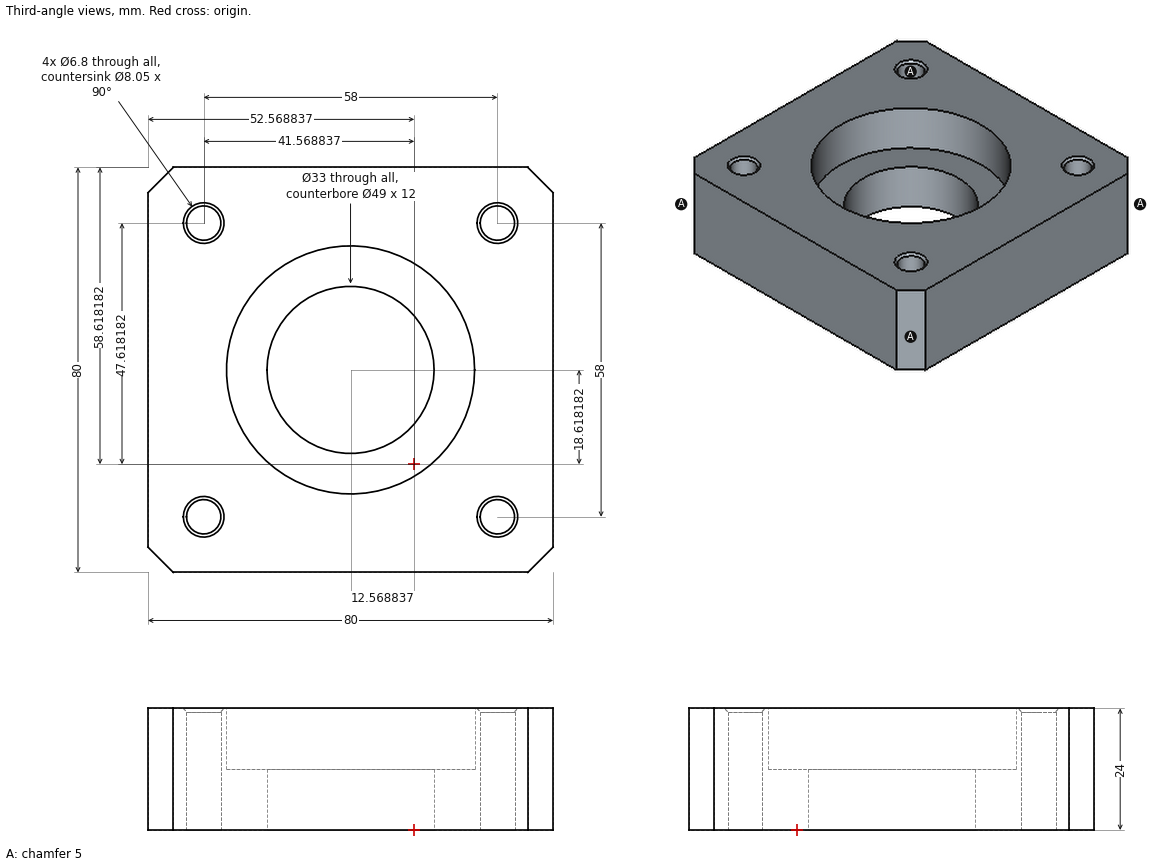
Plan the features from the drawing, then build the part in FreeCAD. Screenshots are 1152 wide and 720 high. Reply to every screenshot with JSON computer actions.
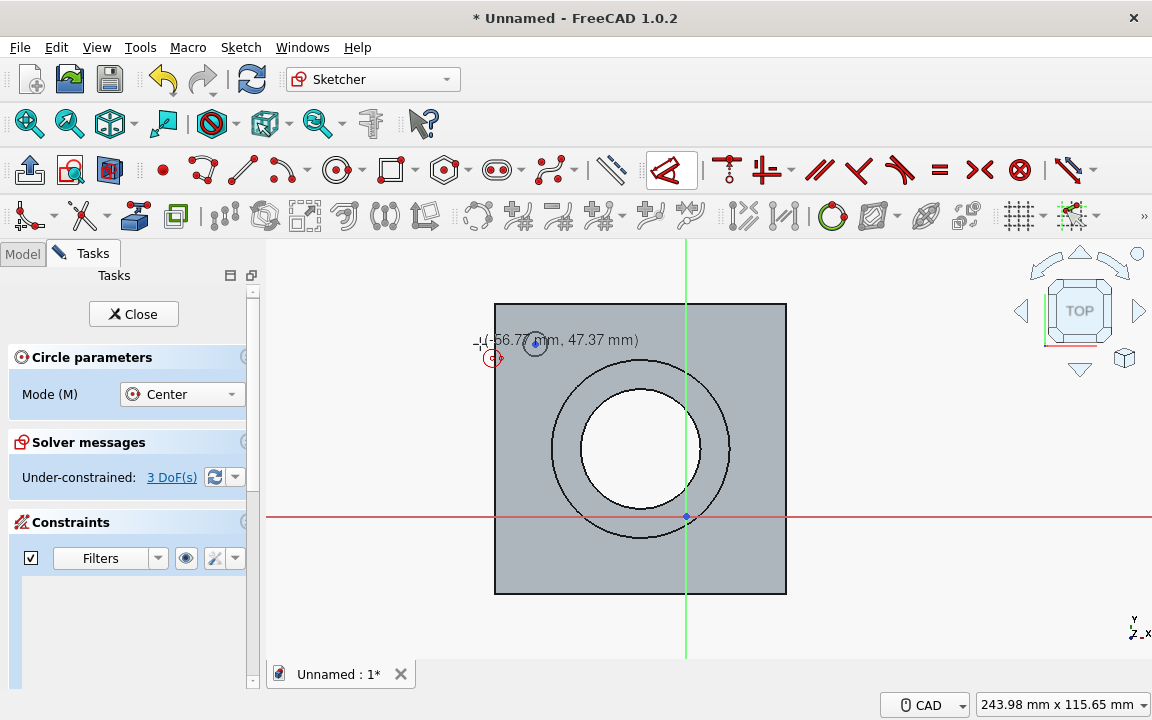
{"action": "scroll", "coordinate": [746, 344], "scroll_direction": "up", "scroll_amount": 4}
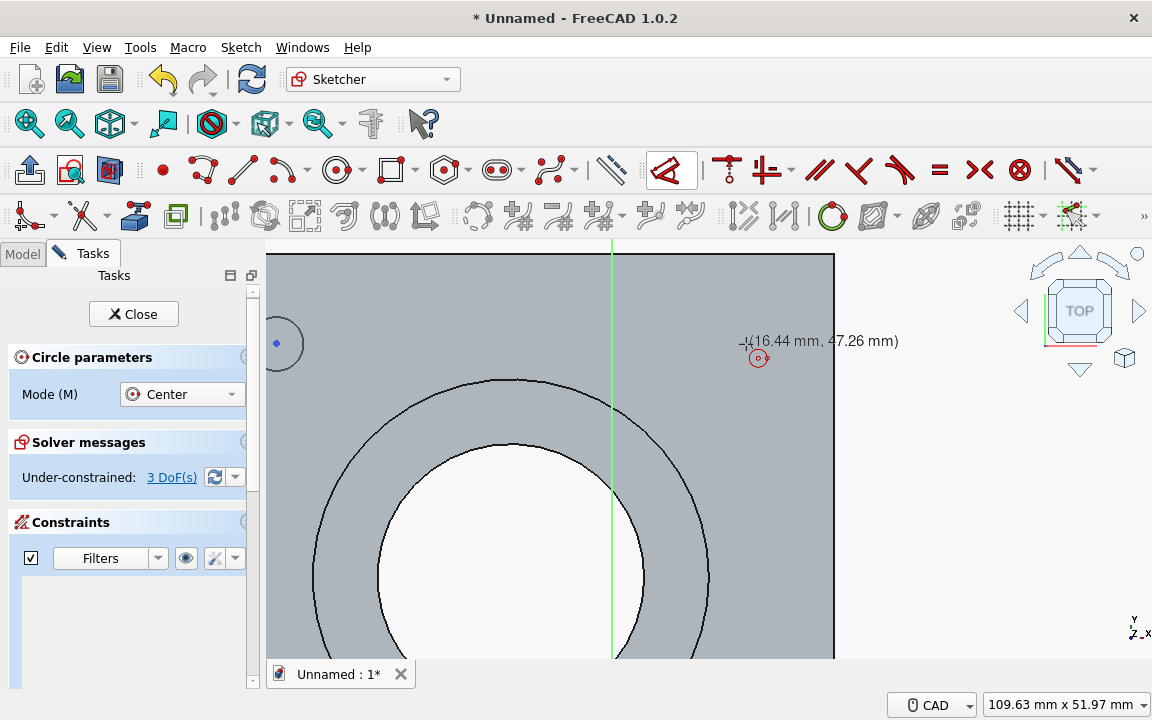
{"action": "left_click", "coordinate": [745, 343]}
{"action": "left_click", "coordinate": [765, 324]}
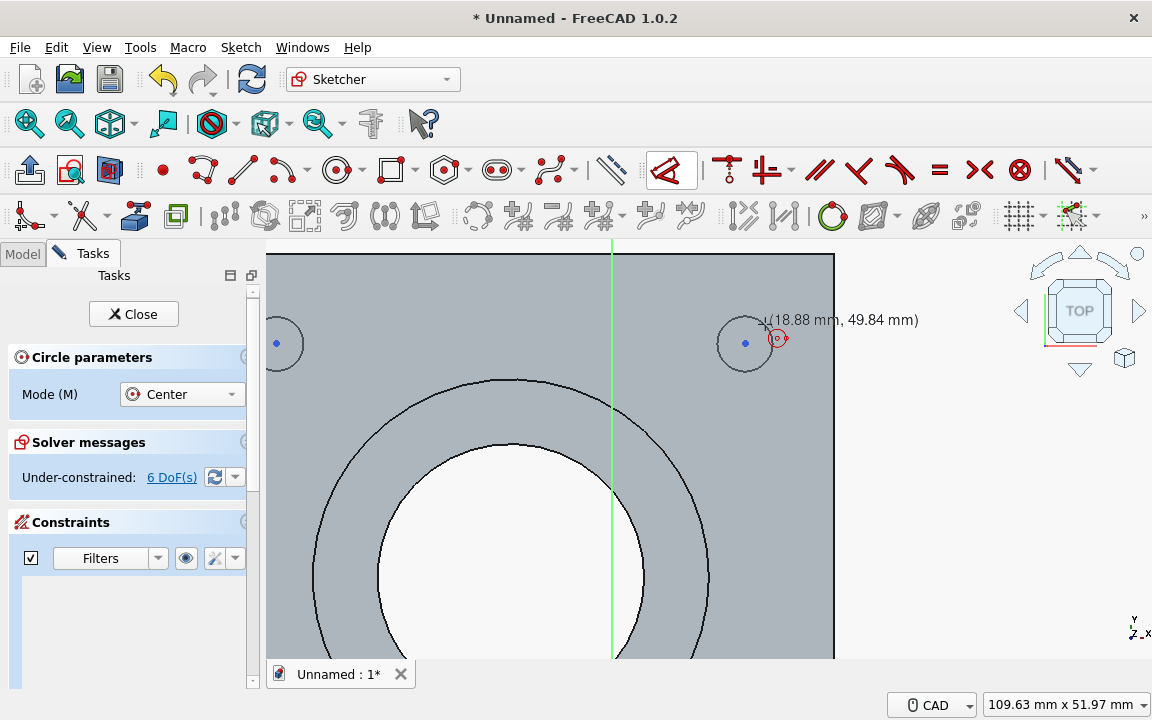
{"action": "scroll", "coordinate": [746, 344], "scroll_direction": "down", "scroll_amount": 4}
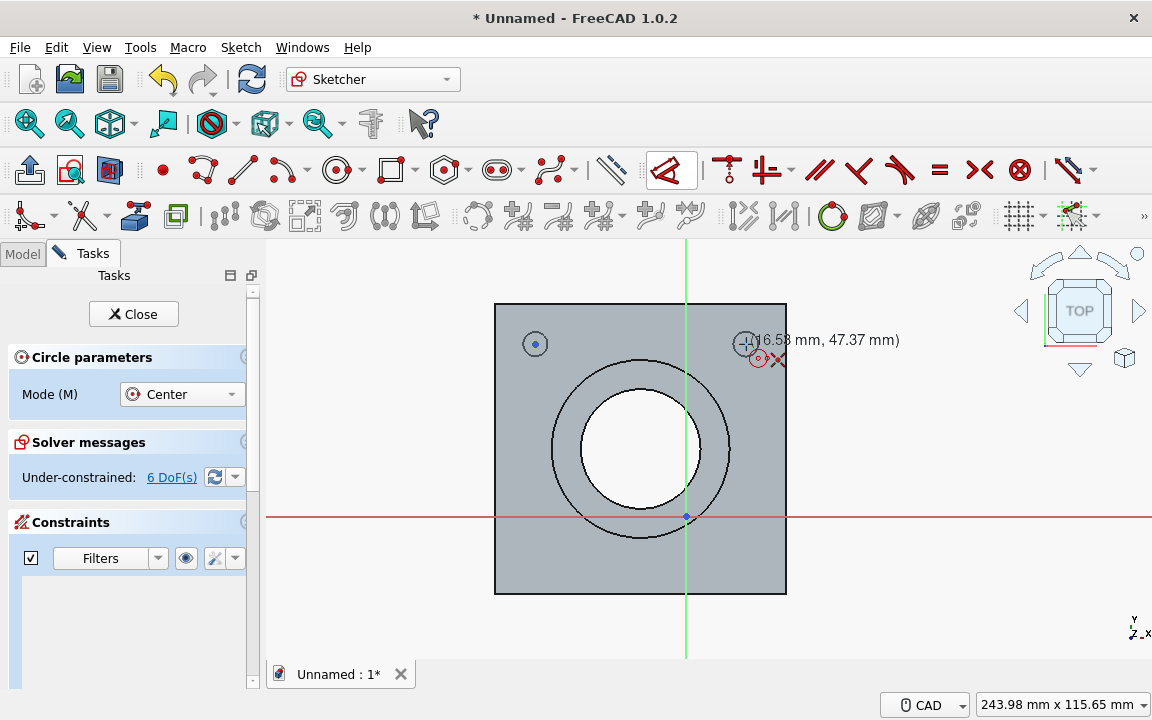
{"action": "scroll", "coordinate": [746, 554], "scroll_direction": "up", "scroll_amount": 4}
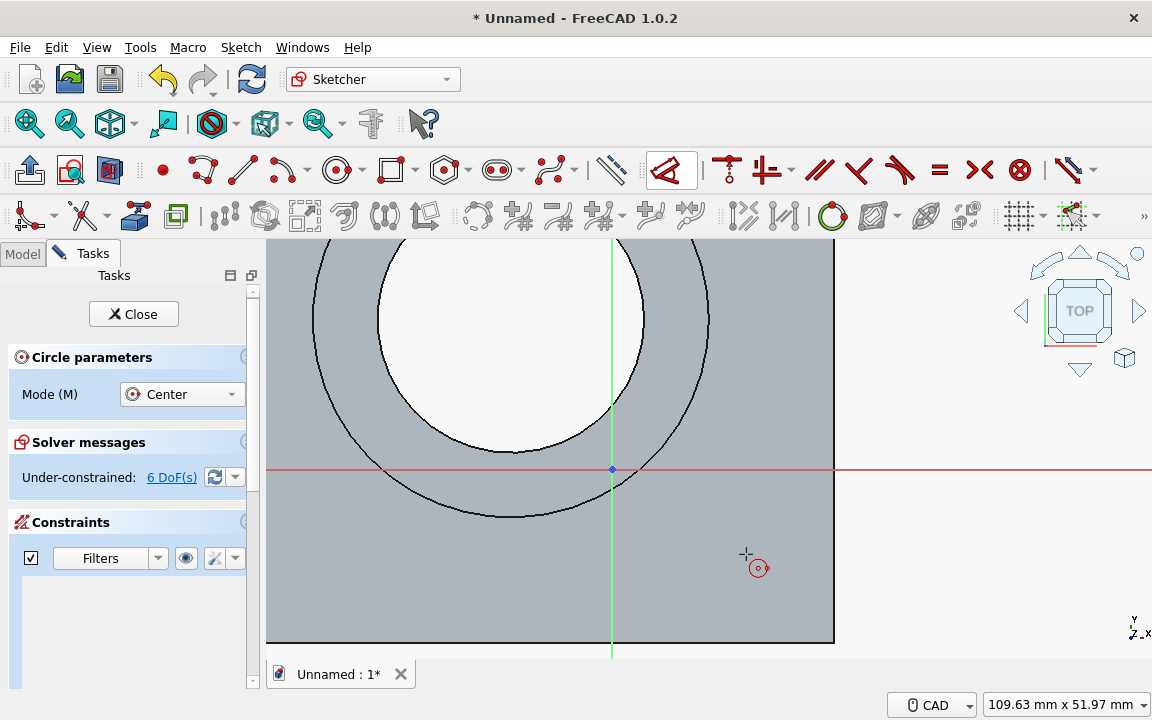
{"action": "left_click", "coordinate": [745, 554]}
{"action": "left_click", "coordinate": [765, 534]}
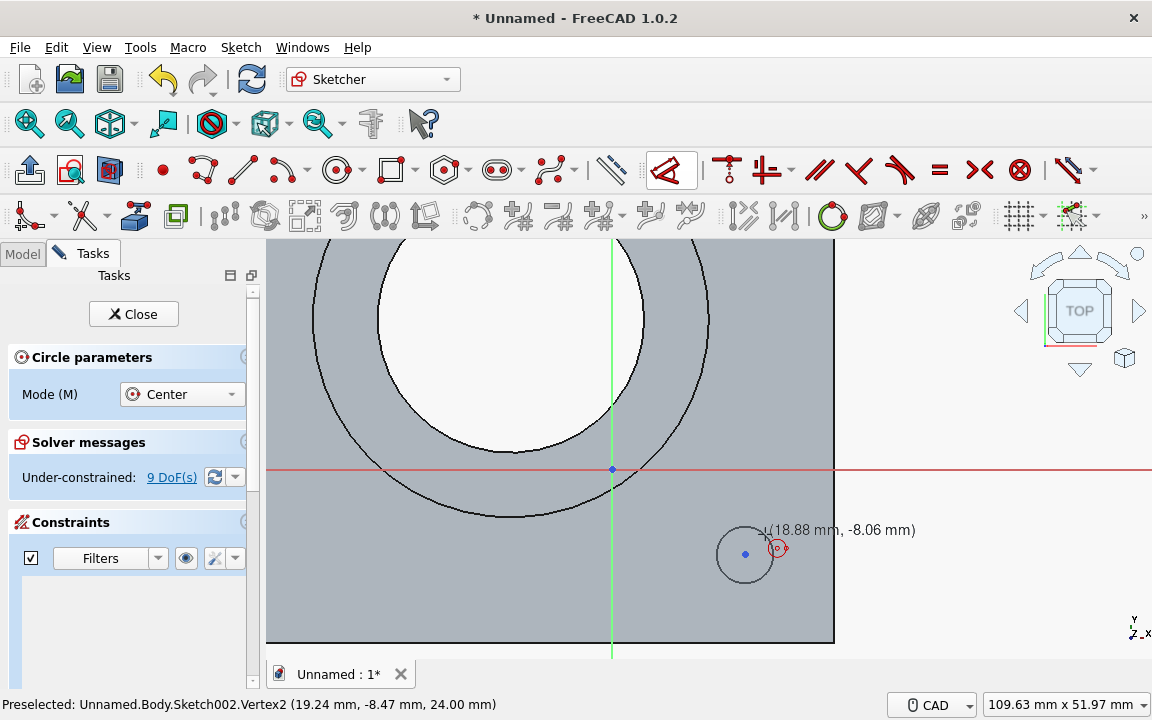
{"action": "scroll", "coordinate": [746, 555], "scroll_direction": "down", "scroll_amount": 4}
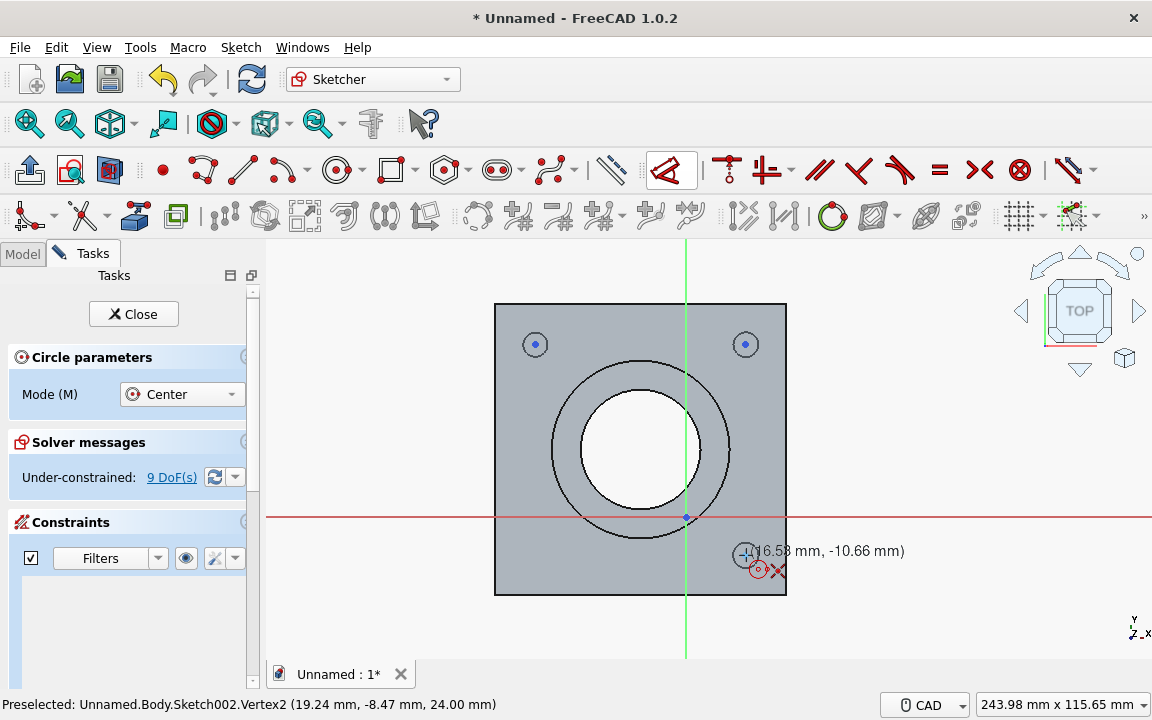
{"action": "scroll", "coordinate": [535, 555], "scroll_direction": "up", "scroll_amount": 4}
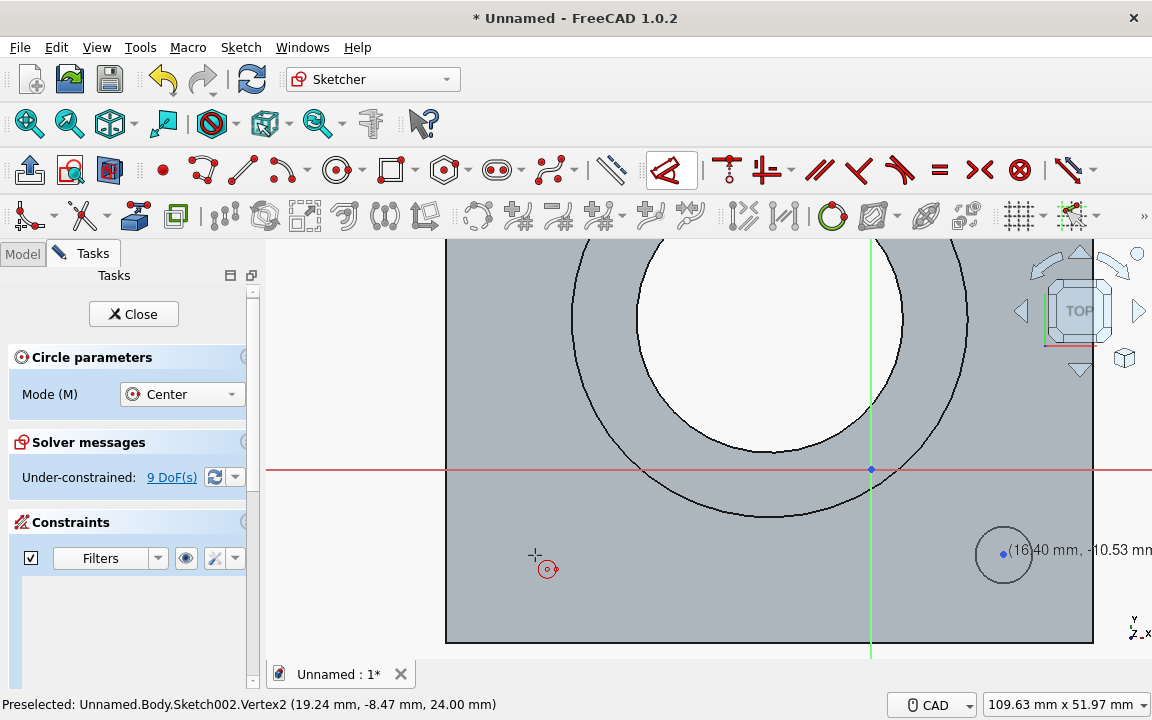
{"action": "left_click", "coordinate": [535, 554]}
{"action": "left_click", "coordinate": [555, 534]}
{"action": "key", "text": "Escape"}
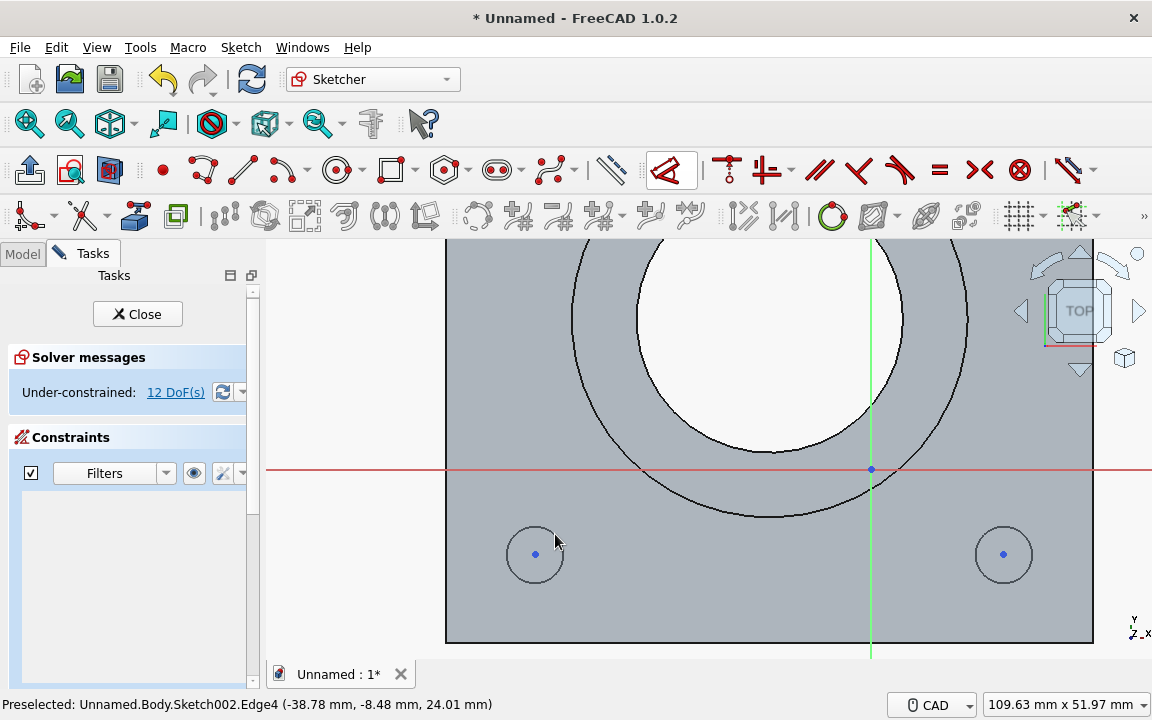
{"action": "scroll", "coordinate": [535, 555], "scroll_direction": "down", "scroll_amount": 4}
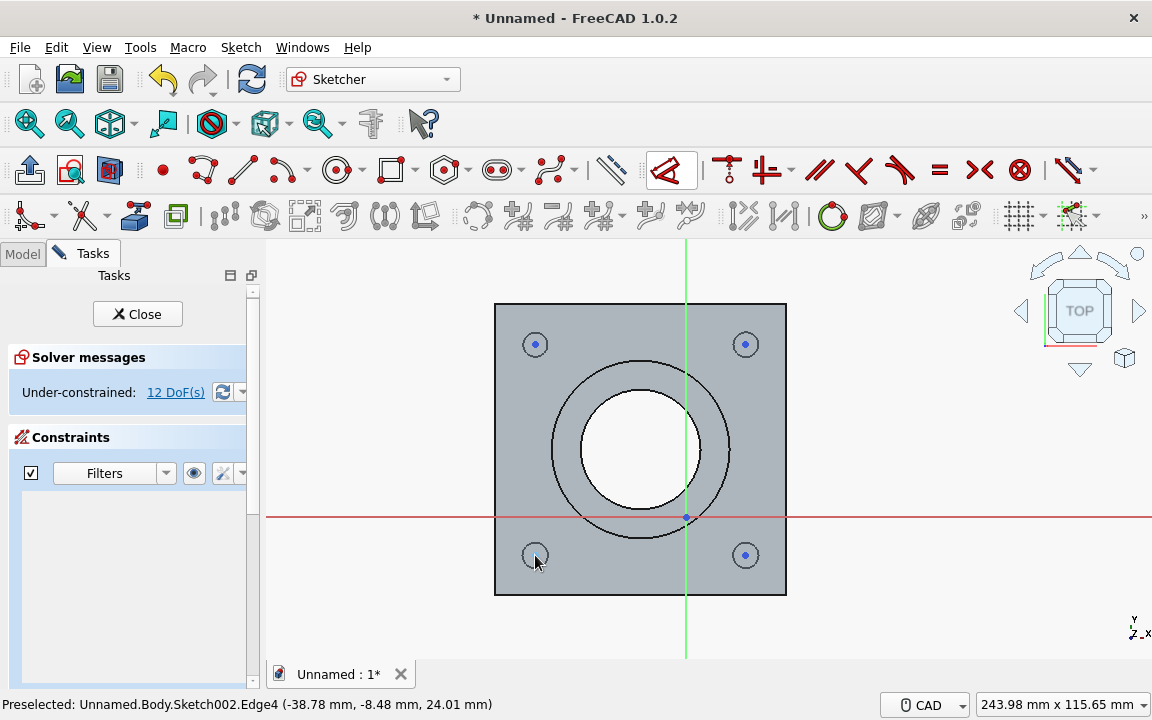
{"action": "left_click", "coordinate": [544, 336]}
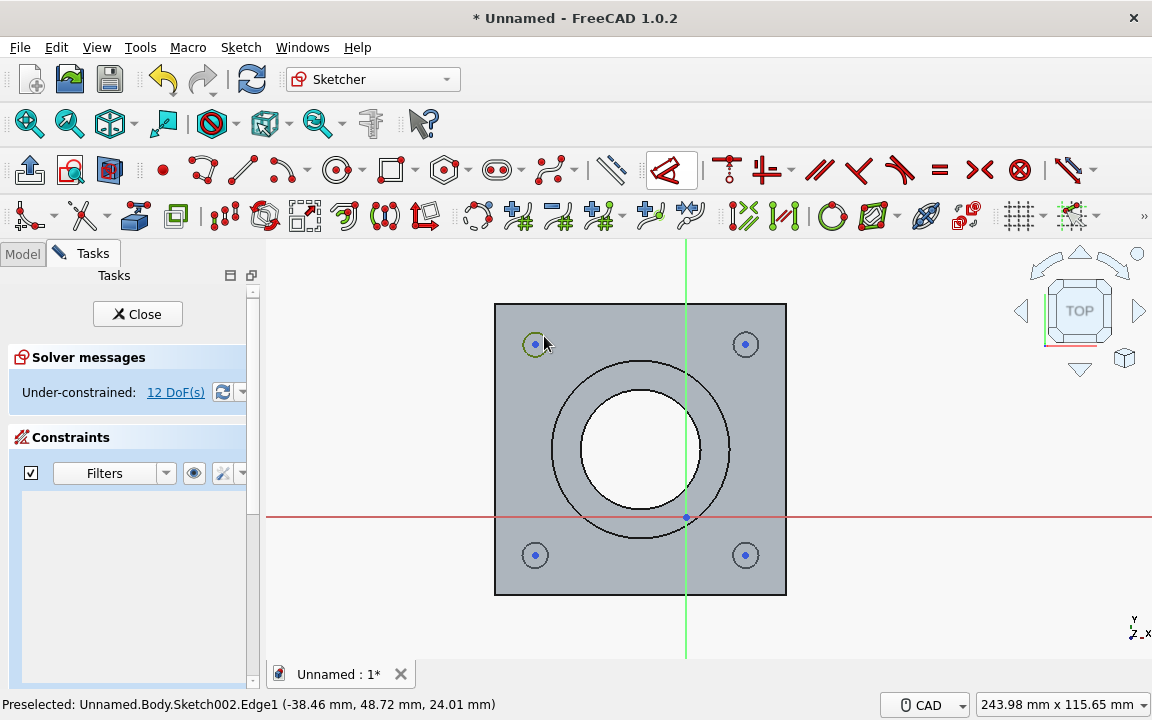
{"action": "left_click", "coordinate": [755, 336]}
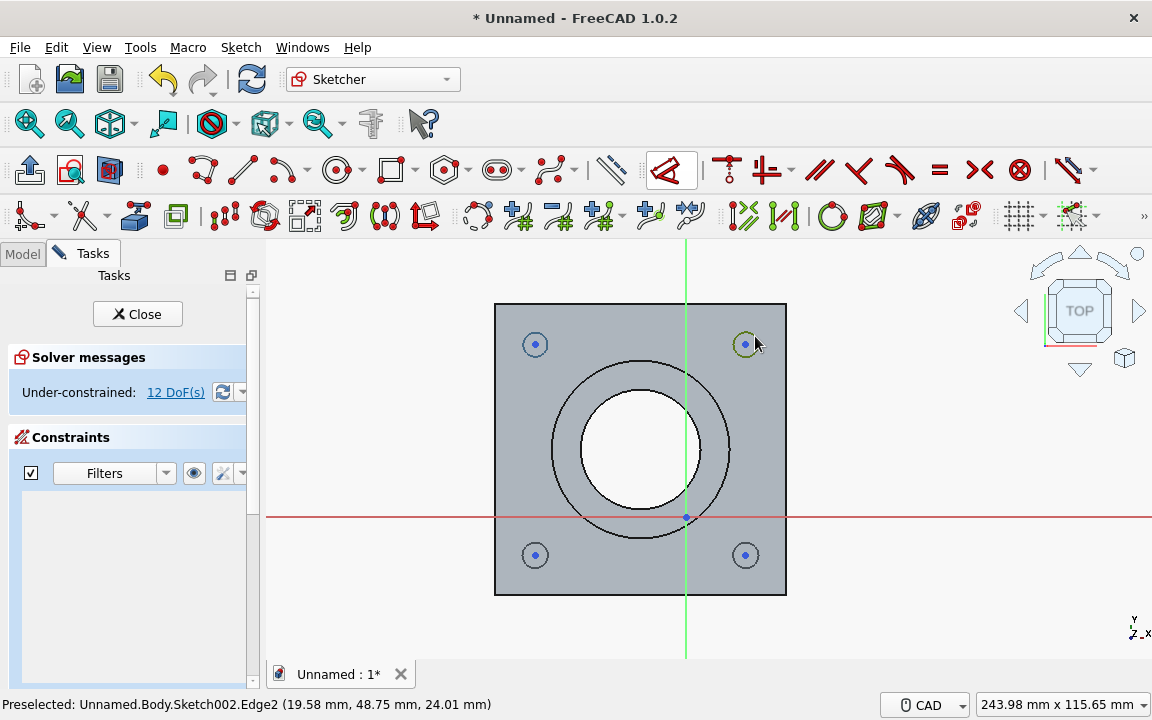
{"action": "left_click", "coordinate": [755, 546]}